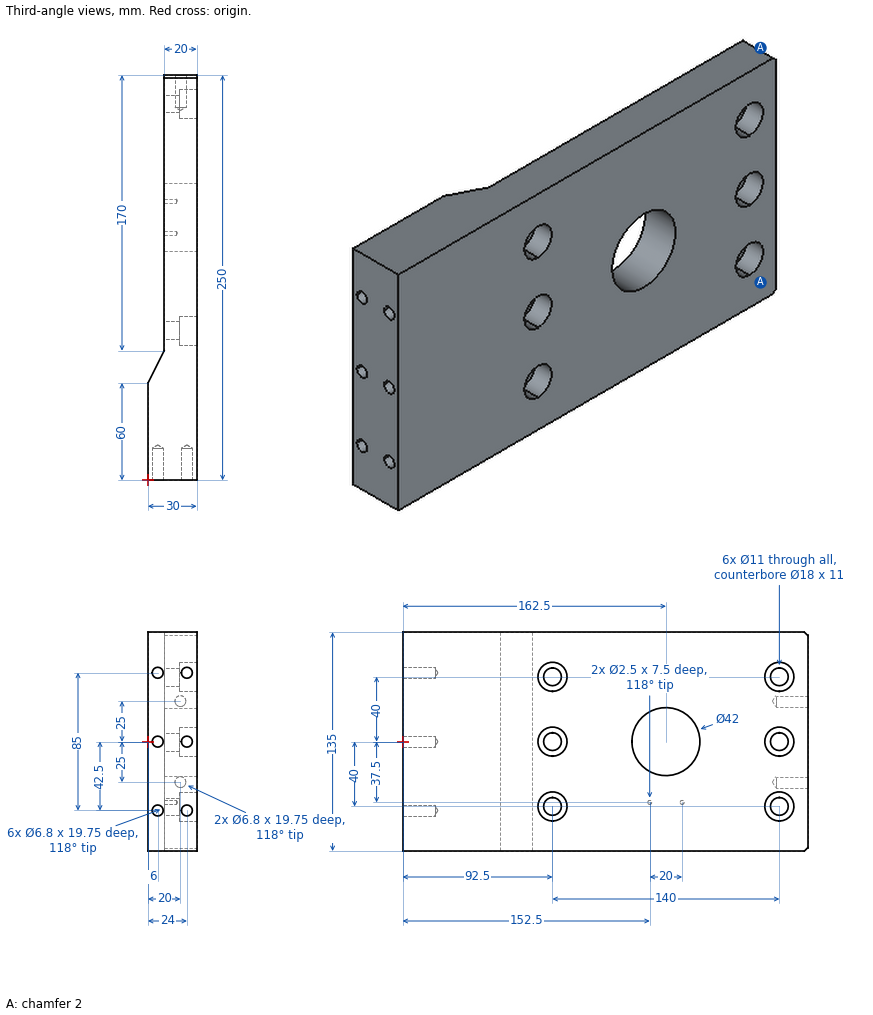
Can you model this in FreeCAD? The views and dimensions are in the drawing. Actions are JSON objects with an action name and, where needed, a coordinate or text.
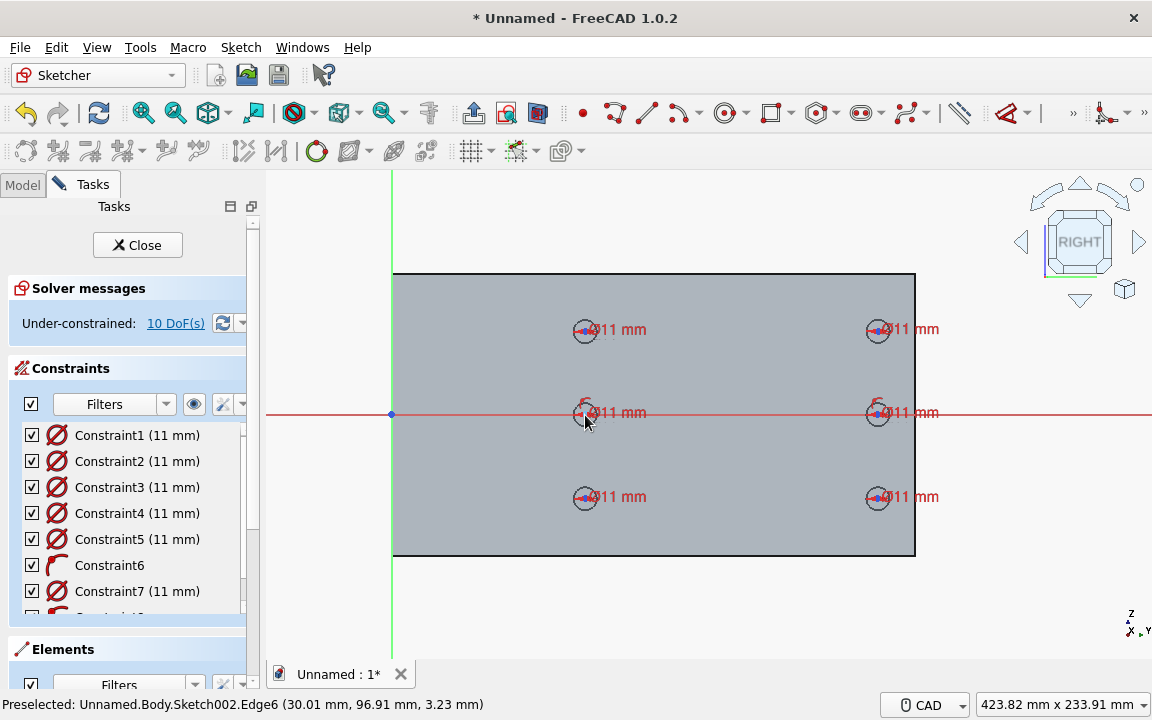
{"action": "left_click", "coordinate": [878, 331]}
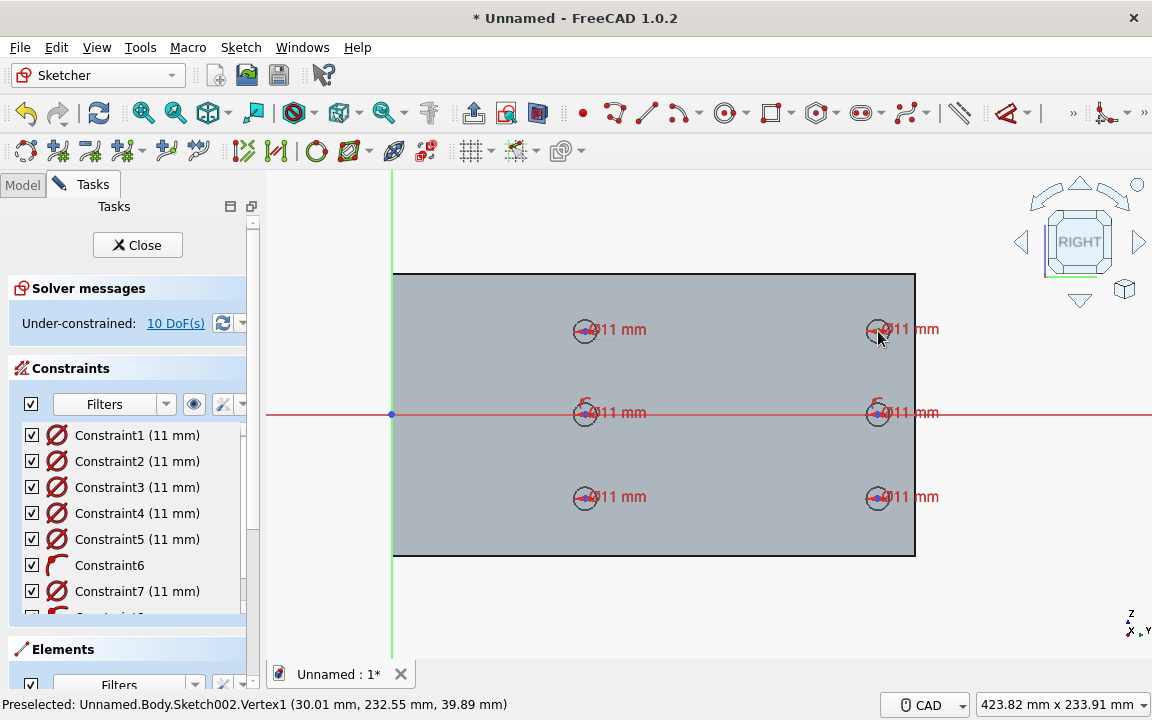
{"action": "left_click", "coordinate": [878, 499]}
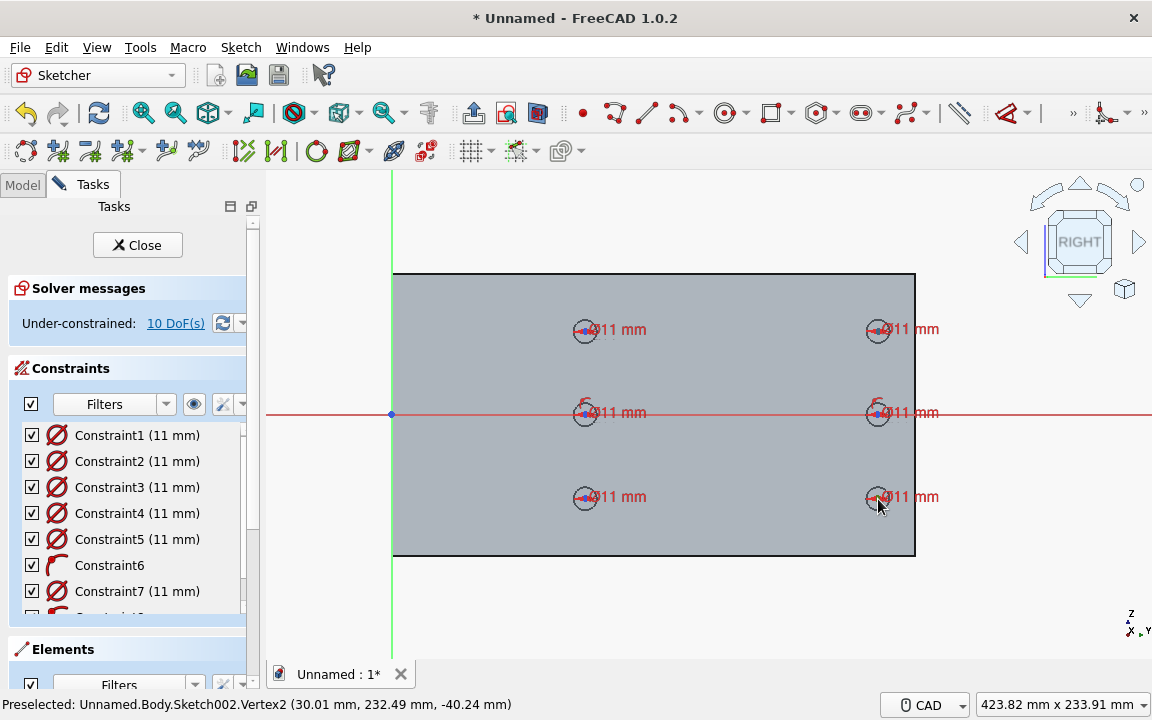
{"action": "key", "text": "v"}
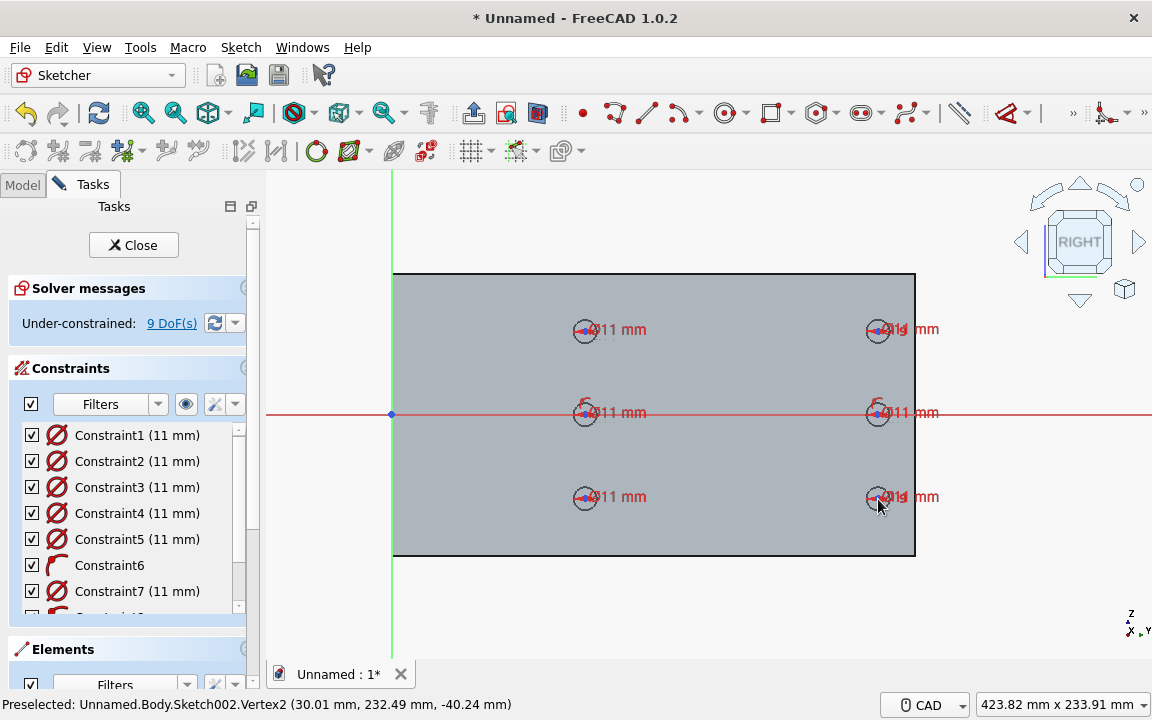
{"action": "left_click", "coordinate": [878, 499]}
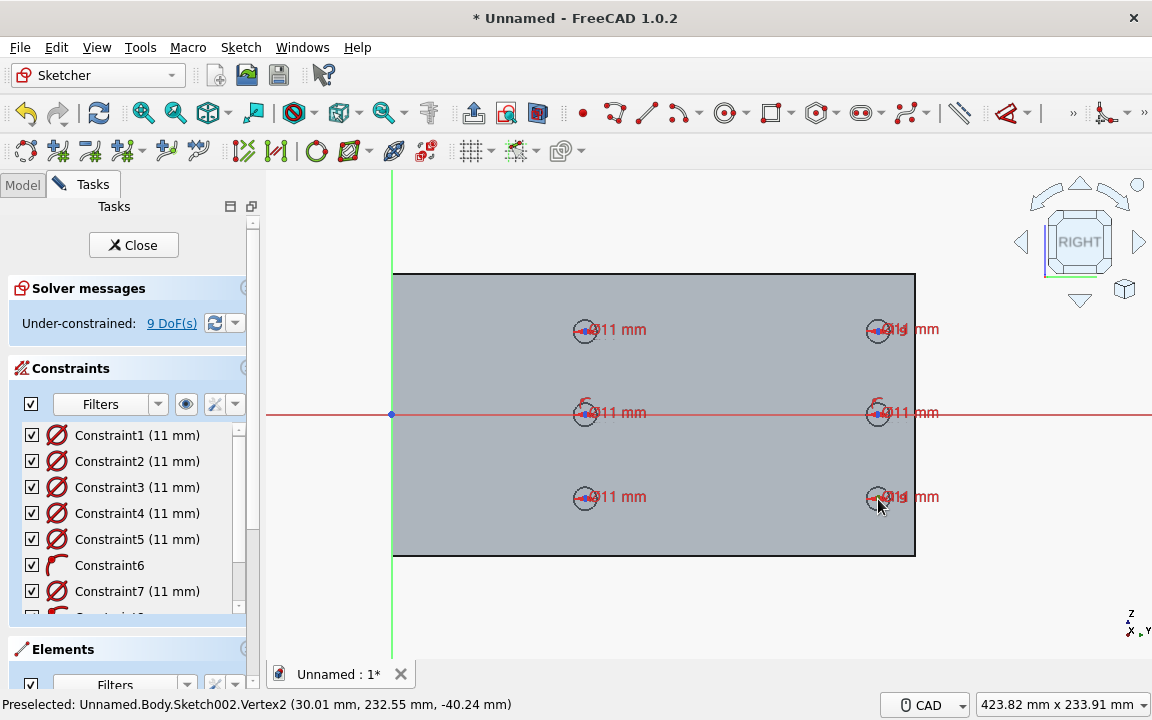
{"action": "left_click", "coordinate": [585, 499]}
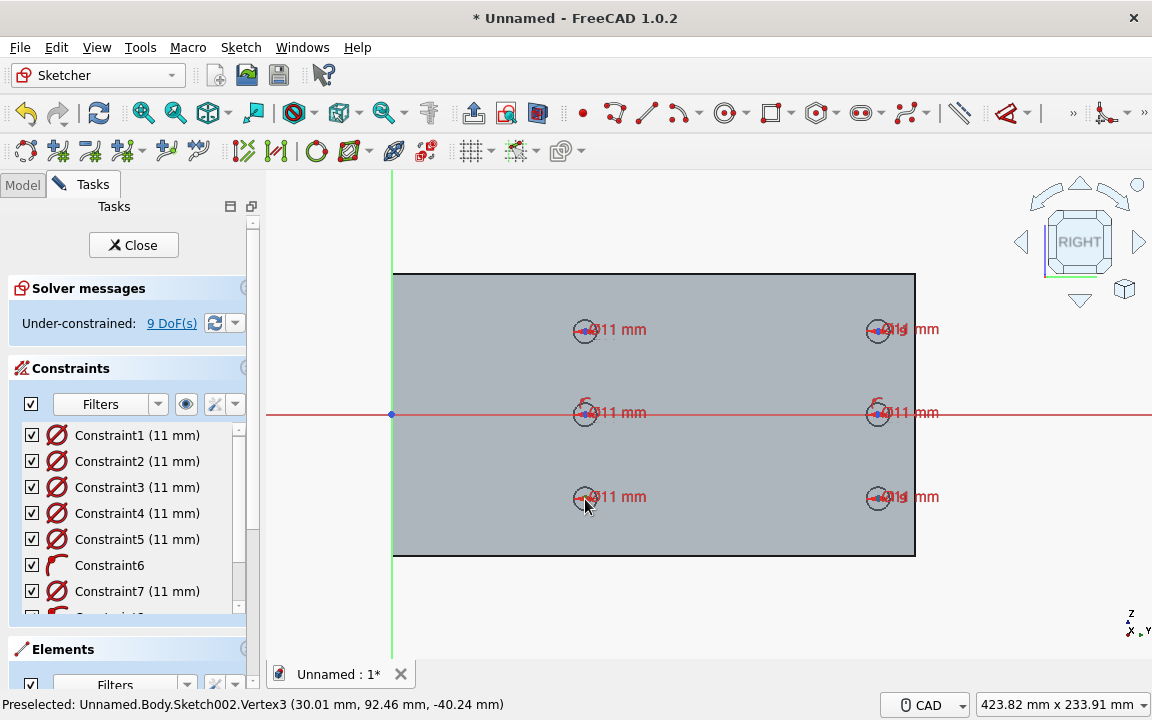
{"action": "key", "text": "h"}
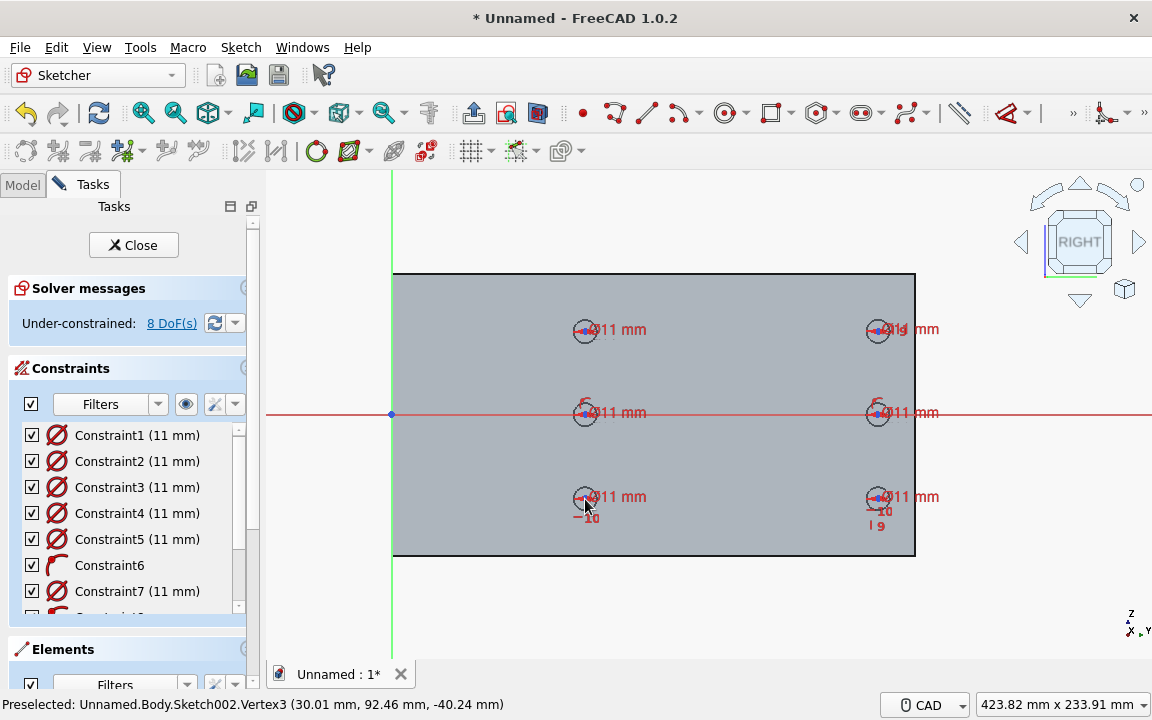
{"action": "left_click", "coordinate": [585, 499]}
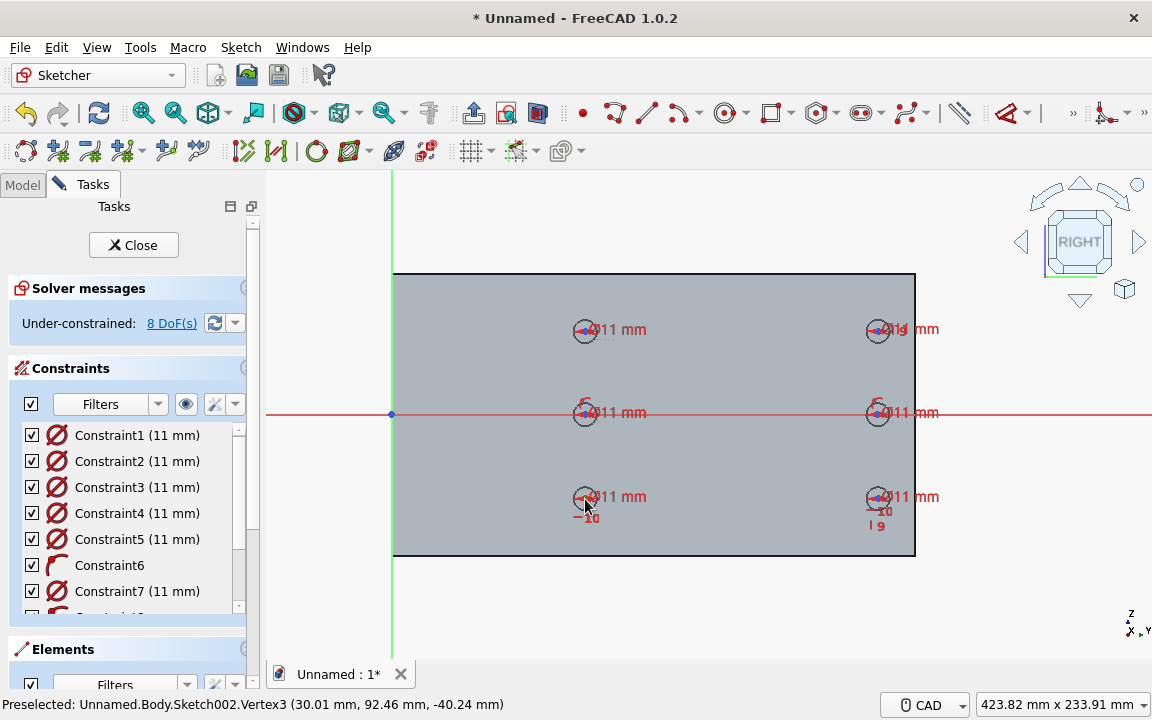
{"action": "left_click", "coordinate": [585, 332]}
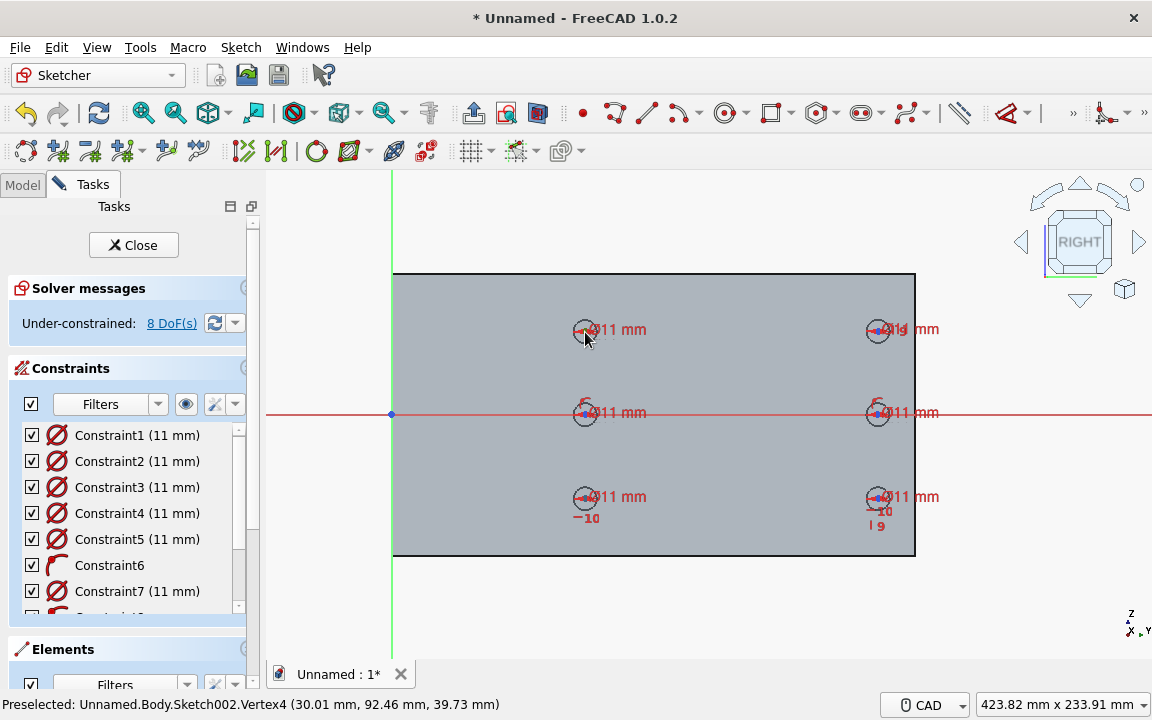
{"action": "key", "text": "v"}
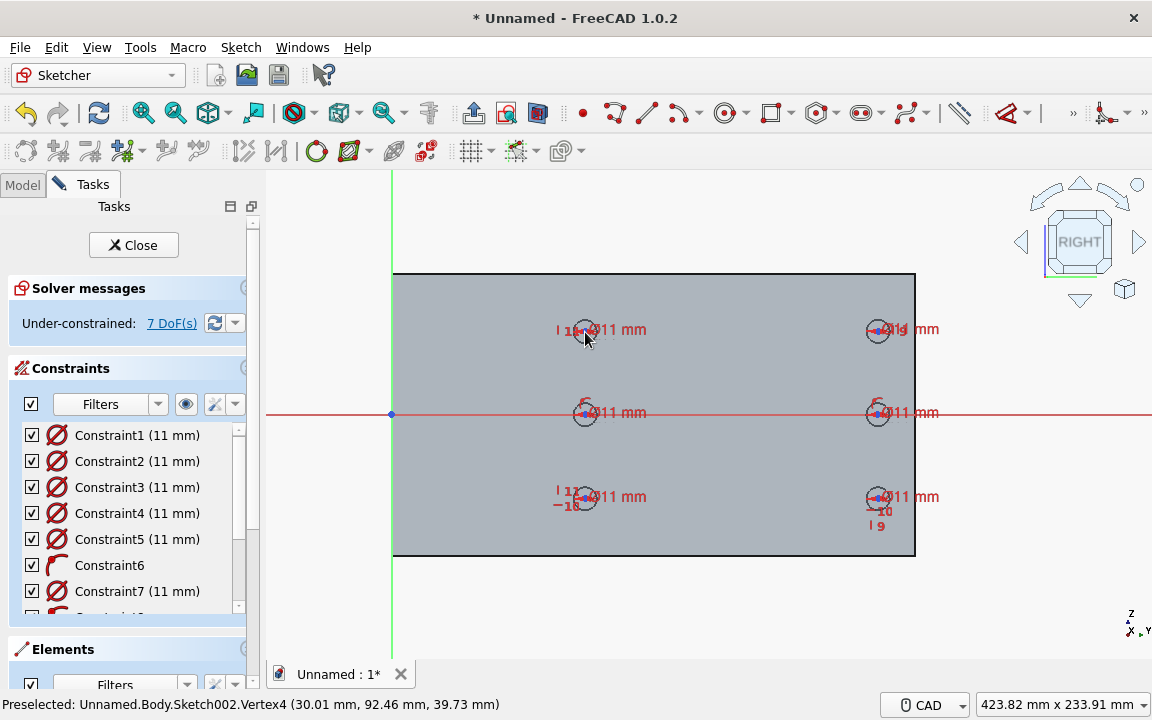
{"action": "left_click", "coordinate": [878, 331]}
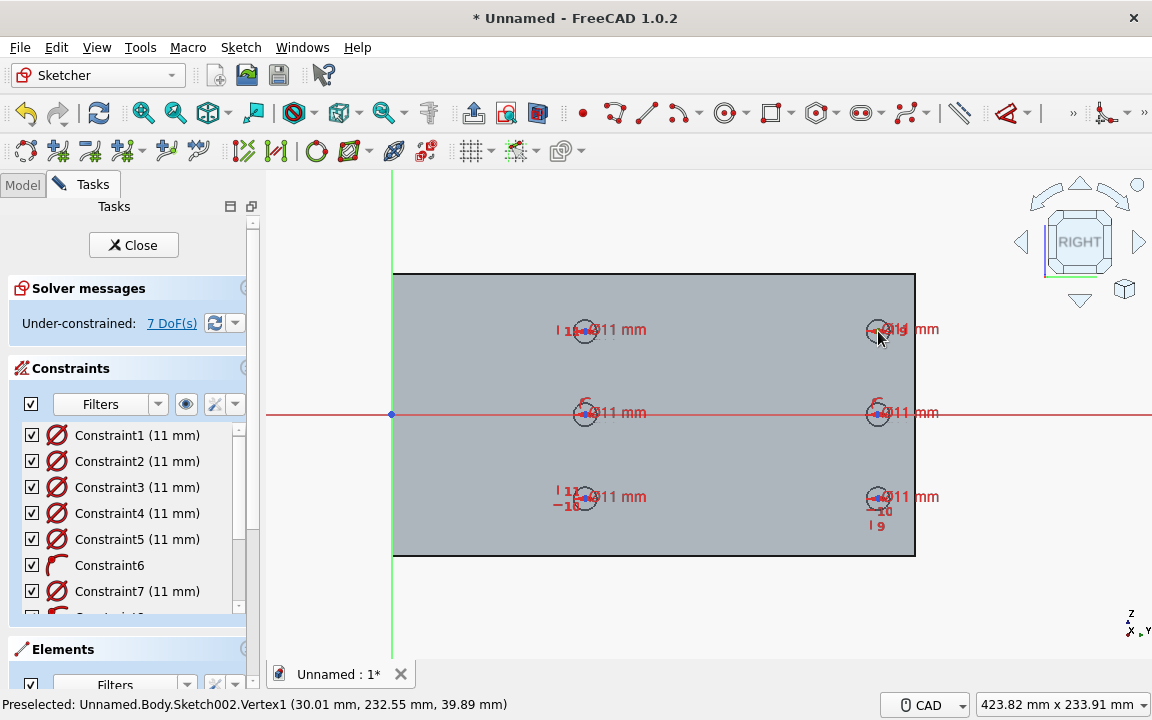
{"action": "left_click", "coordinate": [585, 332]}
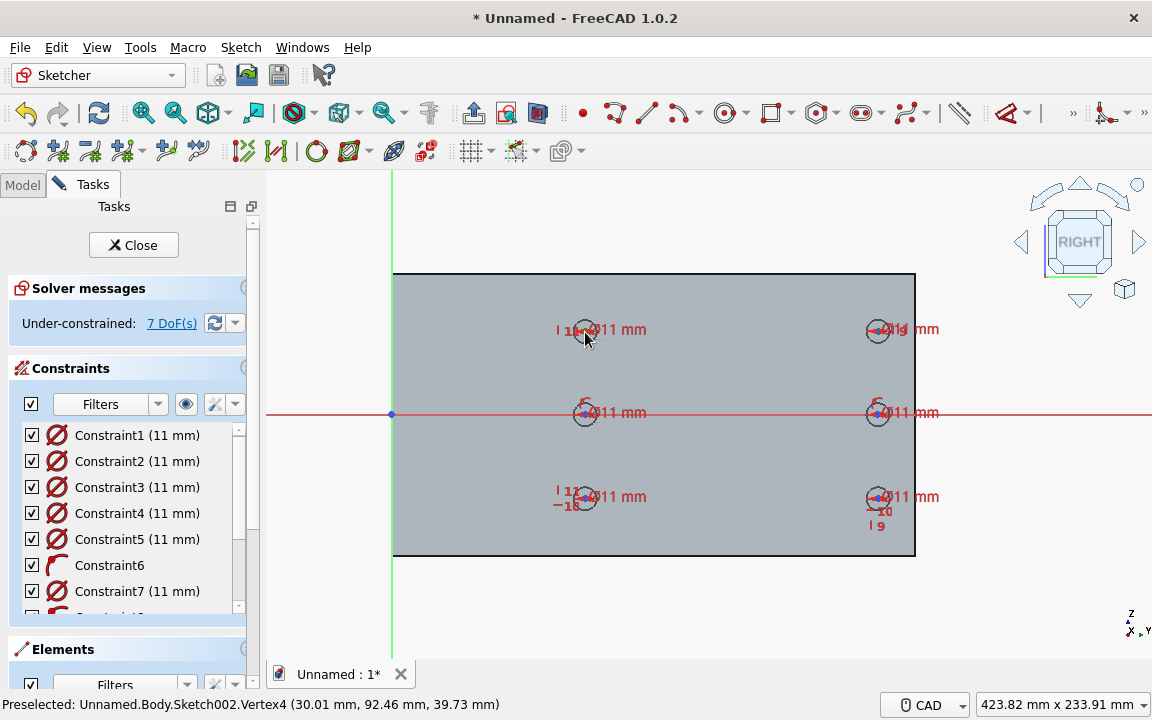
{"action": "key", "text": "h"}